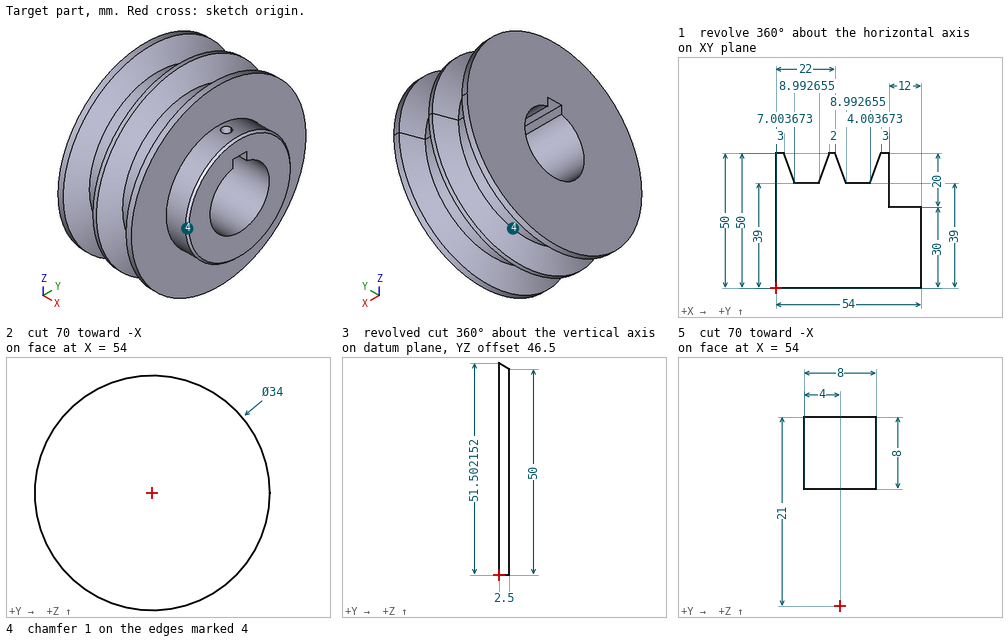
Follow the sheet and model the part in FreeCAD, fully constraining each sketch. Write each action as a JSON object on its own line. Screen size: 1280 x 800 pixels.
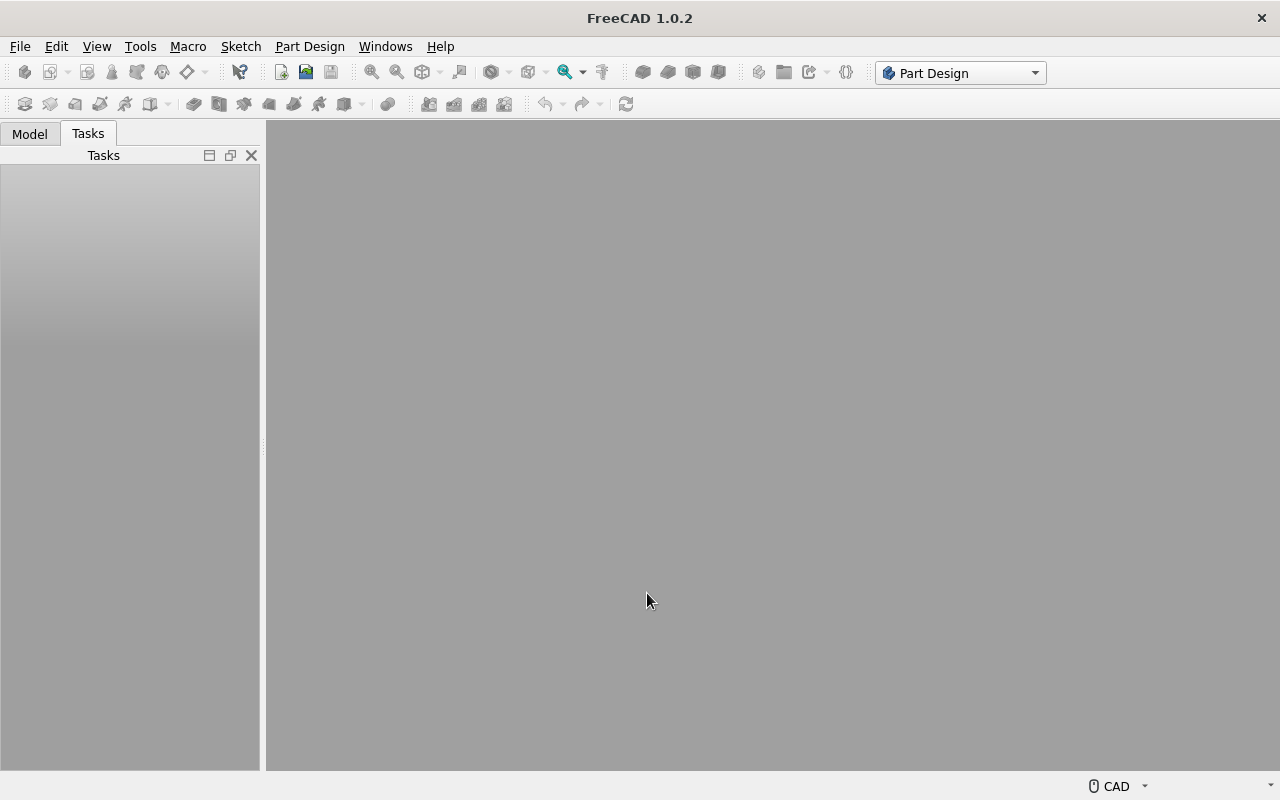
{"action": "left_click", "coordinate": [281, 72]}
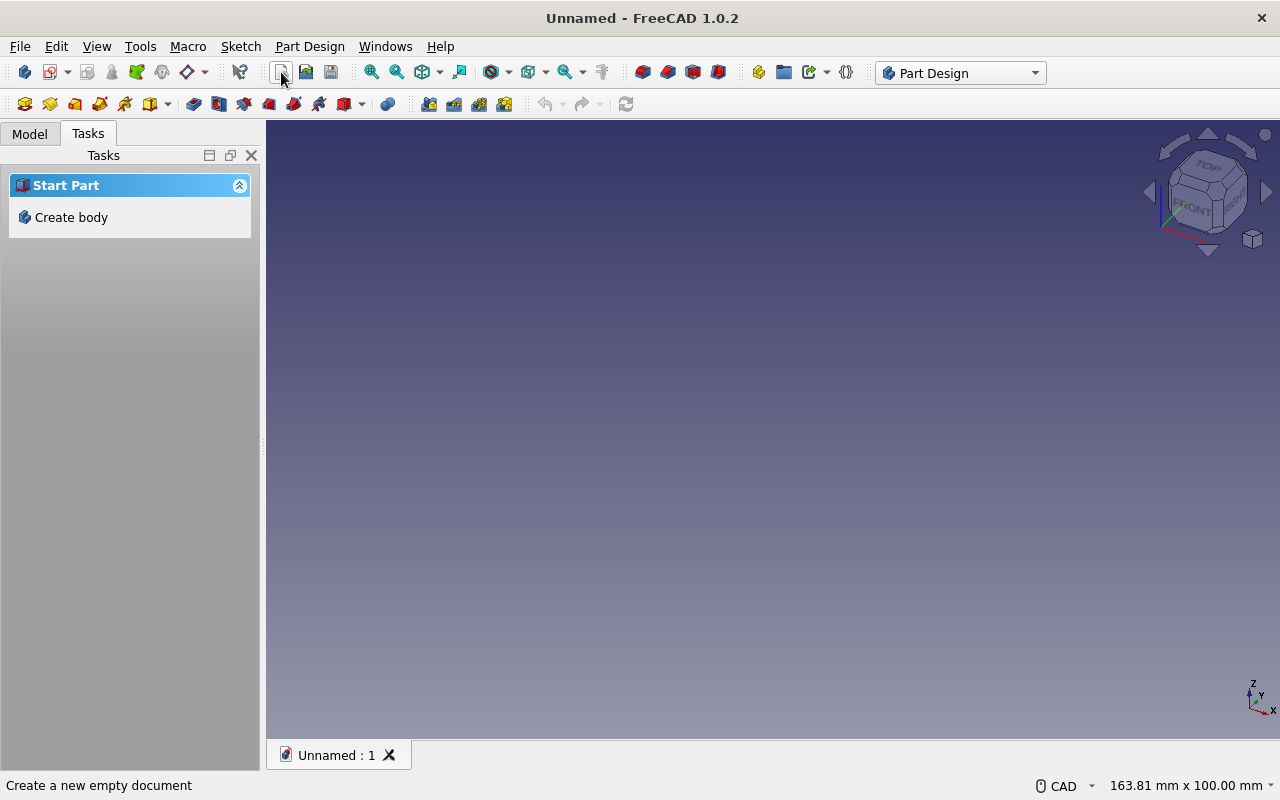
{"action": "left_click", "coordinate": [50, 72]}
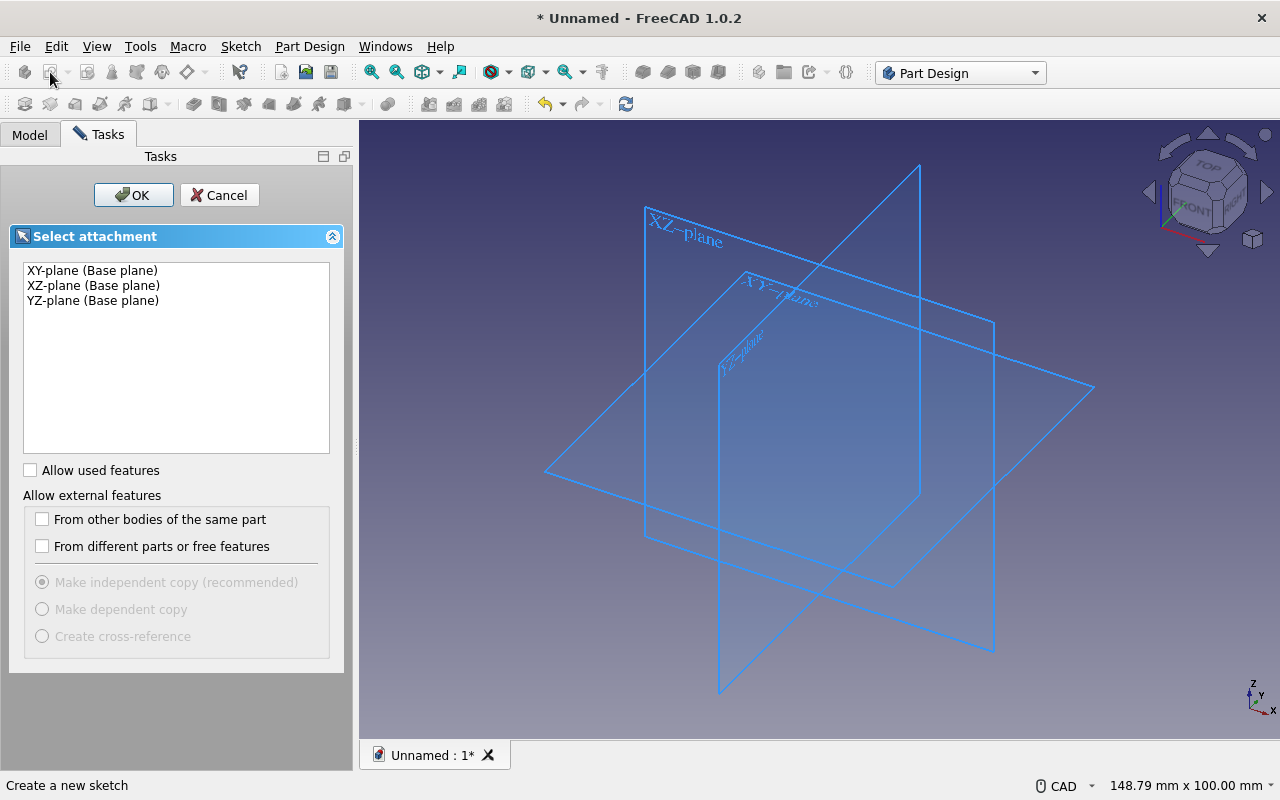
{"action": "left_click", "coordinate": [84, 270]}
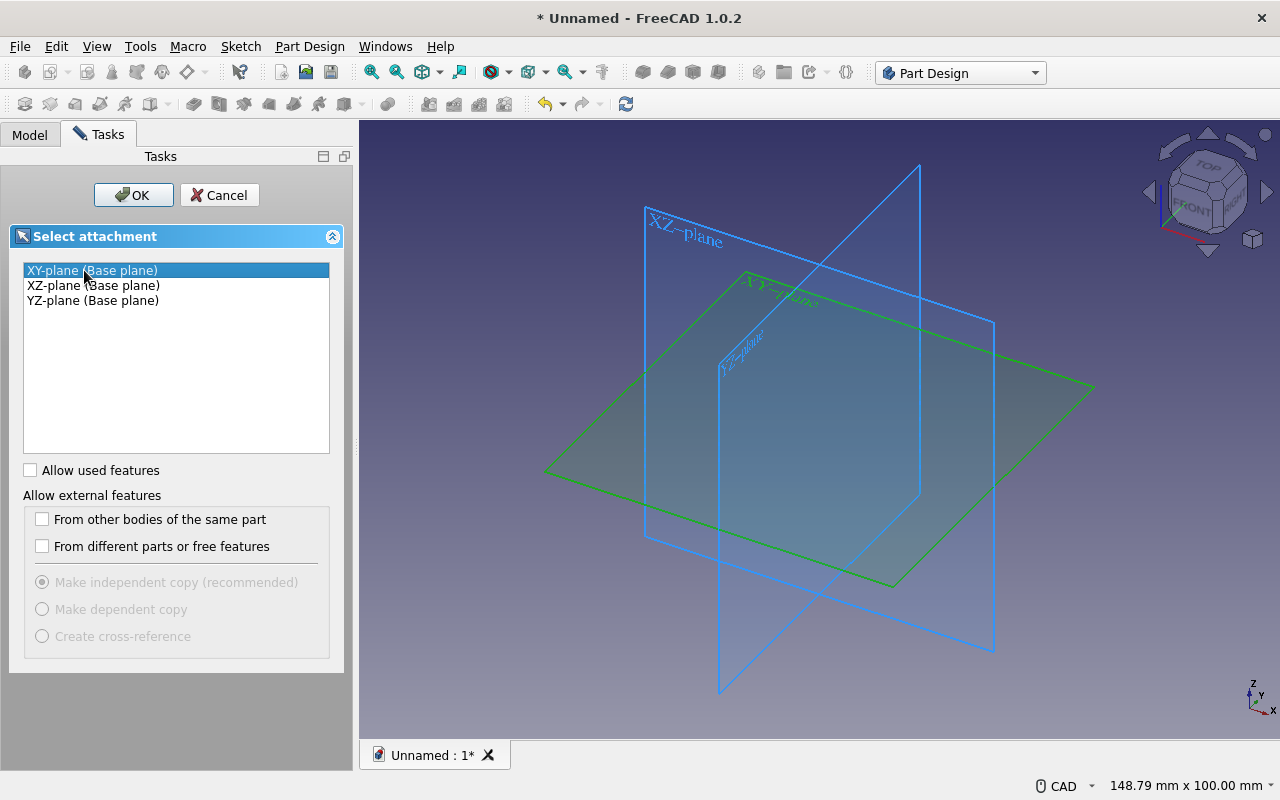
{"action": "left_click", "coordinate": [134, 195]}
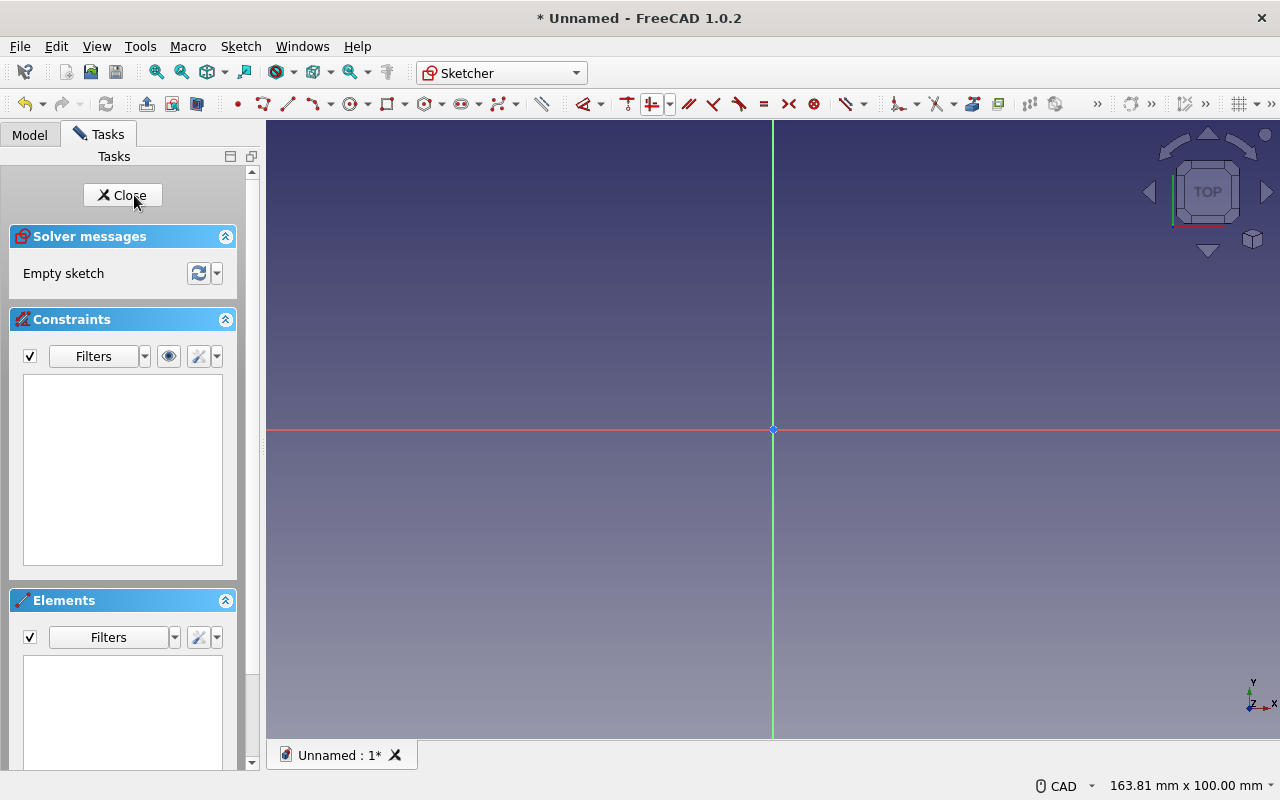
{"action": "scroll", "coordinate": [294, 711], "scroll_direction": "down", "scroll_amount": 1}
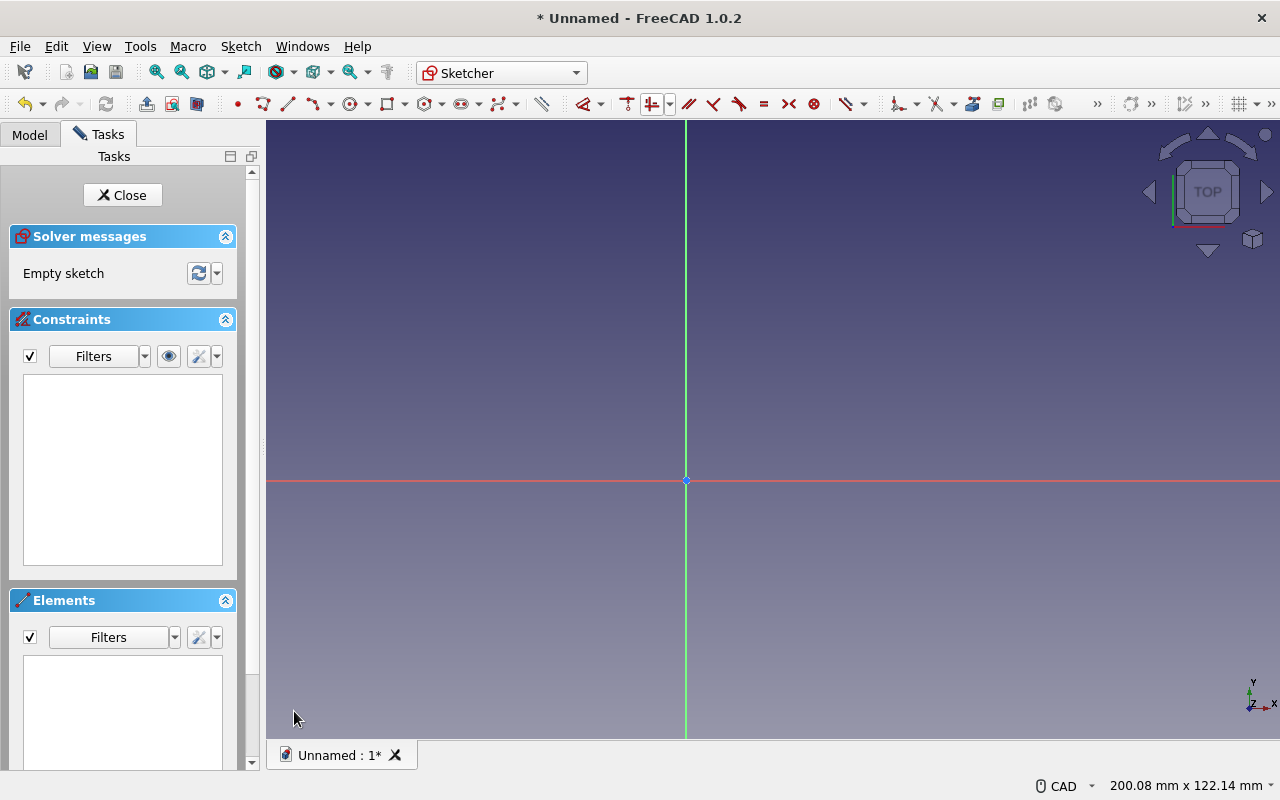
{"action": "scroll", "coordinate": [1064, 200], "scroll_direction": "up", "scroll_amount": 2}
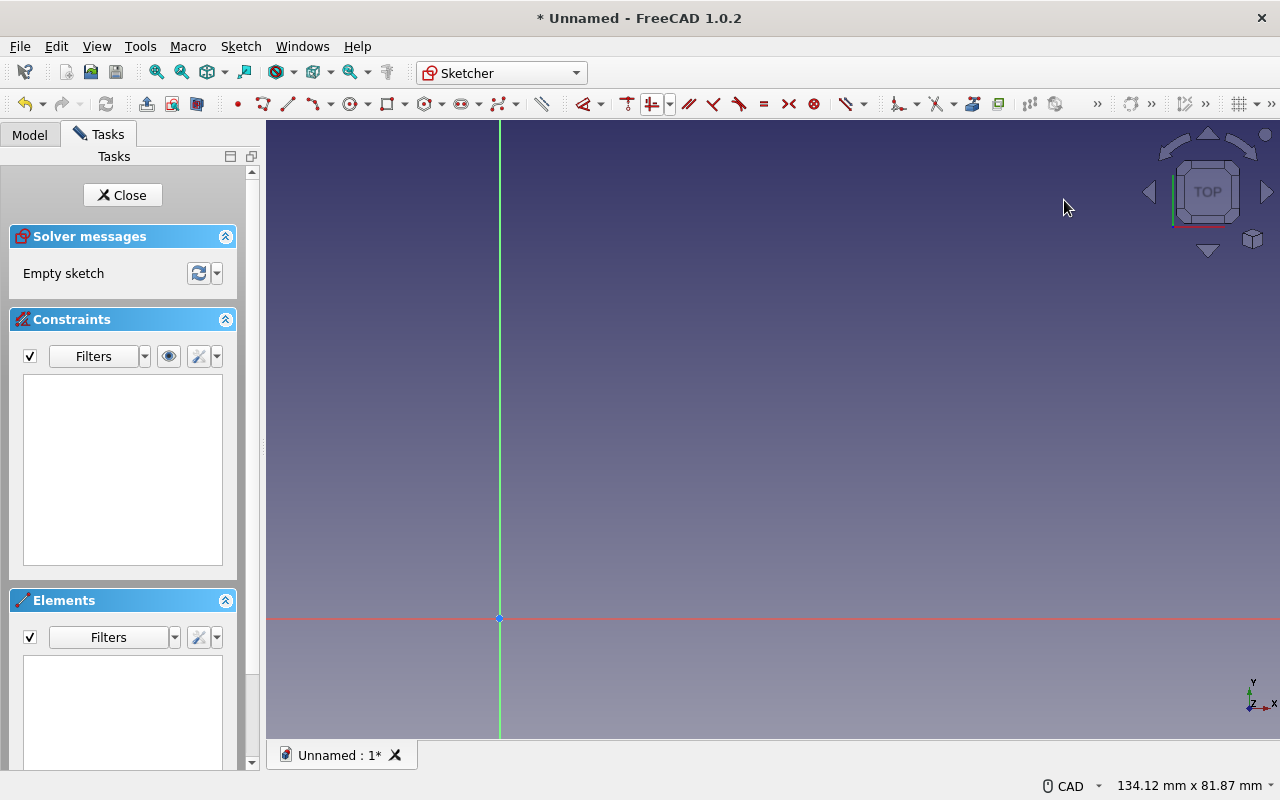
{"action": "left_click", "coordinate": [263, 104]}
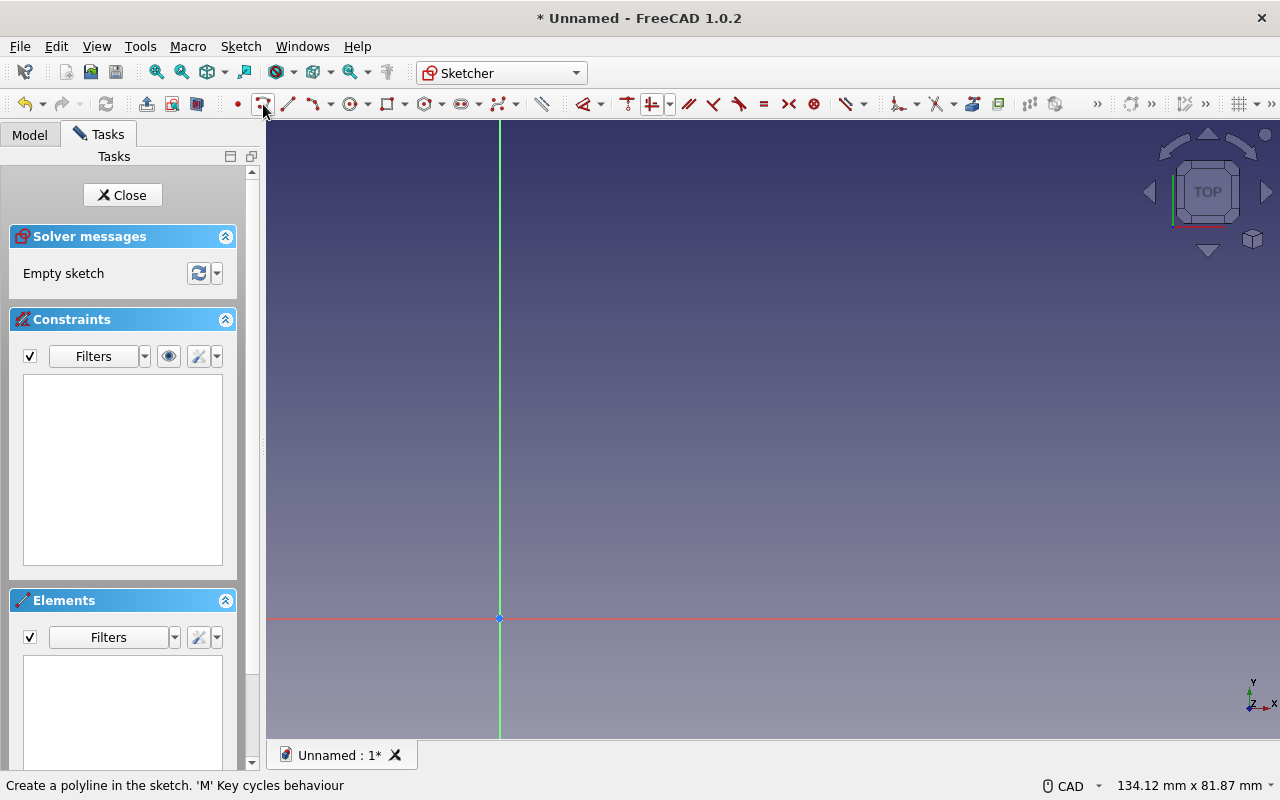
{"action": "left_click", "coordinate": [500, 619]}
{"action": "left_click", "coordinate": [908, 610]}
{"action": "left_click", "coordinate": [908, 392]}
{"action": "left_click", "coordinate": [818, 392]}
{"action": "left_click", "coordinate": [818, 241]}
{"action": "left_click", "coordinate": [795, 241]}
{"action": "left_click", "coordinate": [765, 324]}
{"action": "left_click", "coordinate": [697, 324]}
{"action": "left_click", "coordinate": [666, 241]}
{"action": "left_click", "coordinate": [651, 241]}
{"action": "left_click", "coordinate": [621, 324]}
{"action": "left_click", "coordinate": [553, 324]}
{"action": "left_click", "coordinate": [523, 241]}
{"action": "left_click", "coordinate": [509, 241]}
{"action": "left_click", "coordinate": [500, 619]}
{"action": "key", "text": "Escape"}
{"action": "key", "text": "Escape"}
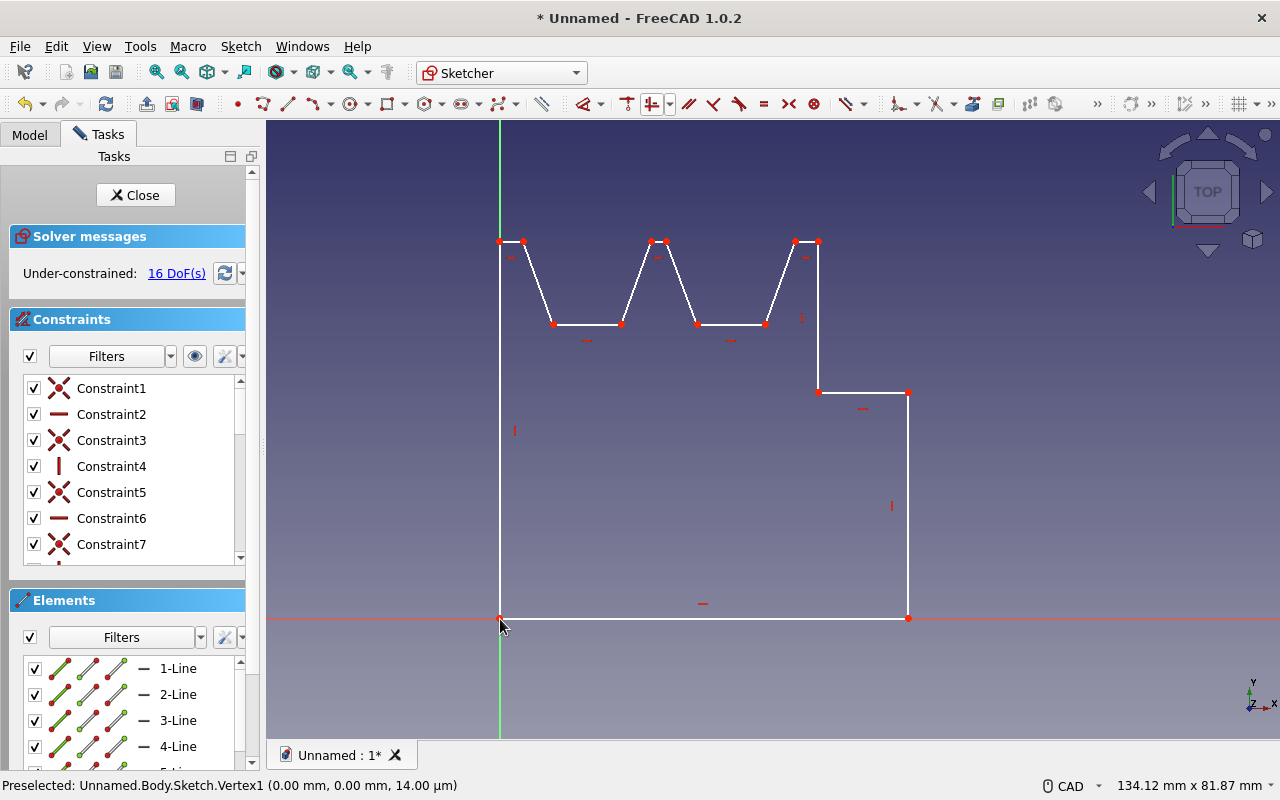
{"action": "key", "text": "d"}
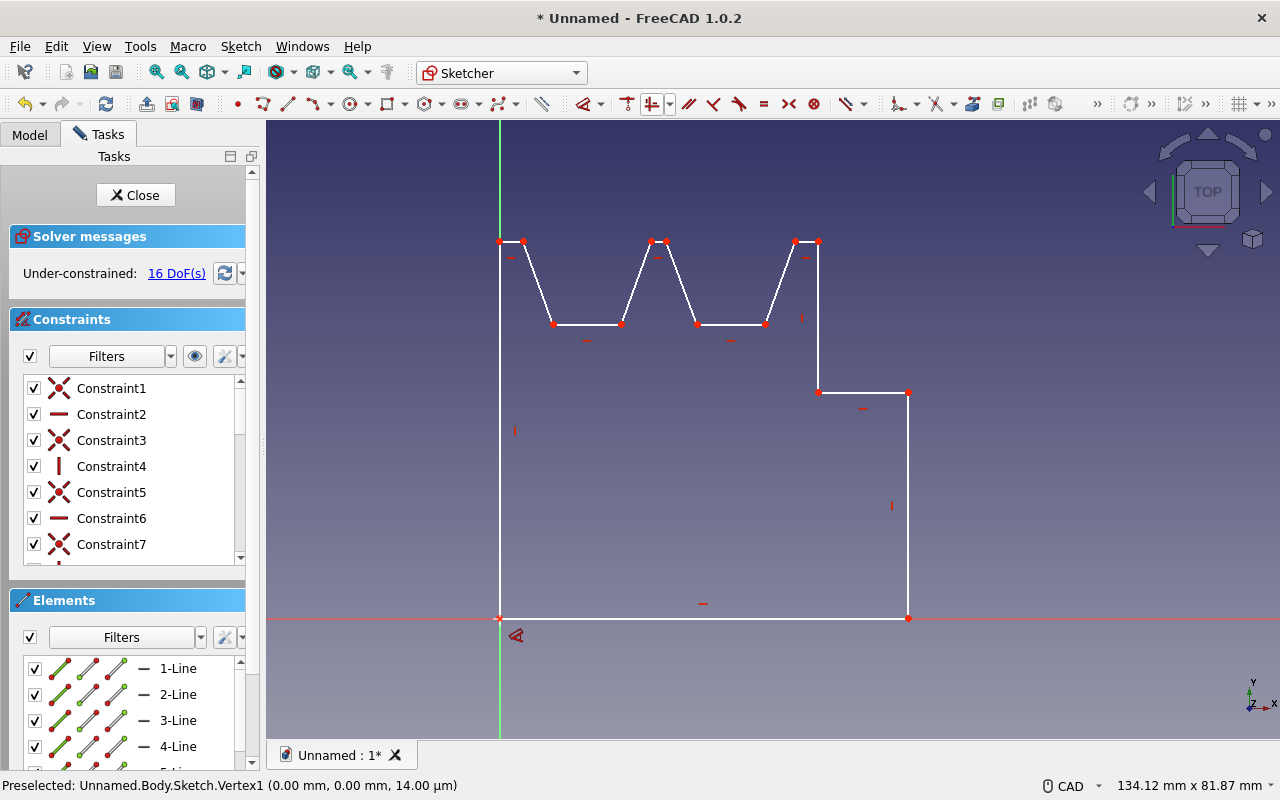
{"action": "scroll", "coordinate": [809, 242], "scroll_direction": "up", "scroll_amount": 3}